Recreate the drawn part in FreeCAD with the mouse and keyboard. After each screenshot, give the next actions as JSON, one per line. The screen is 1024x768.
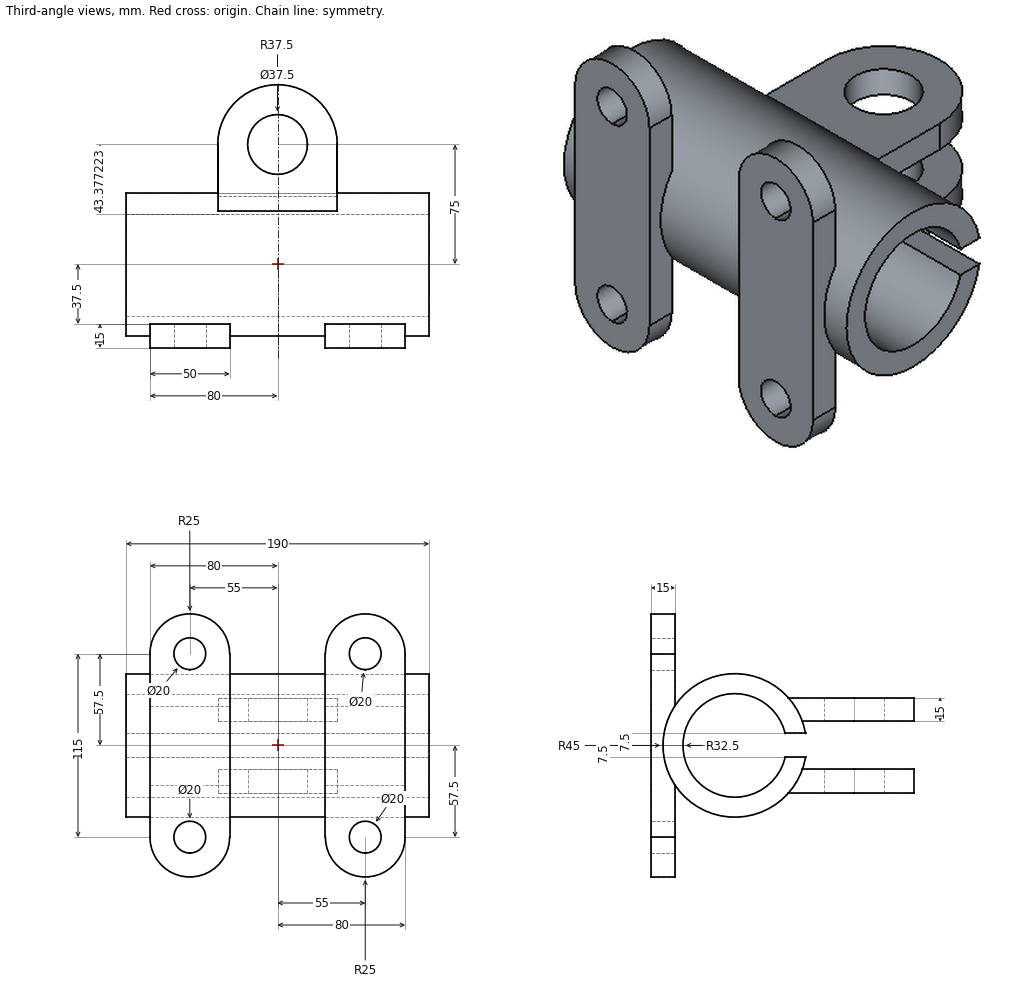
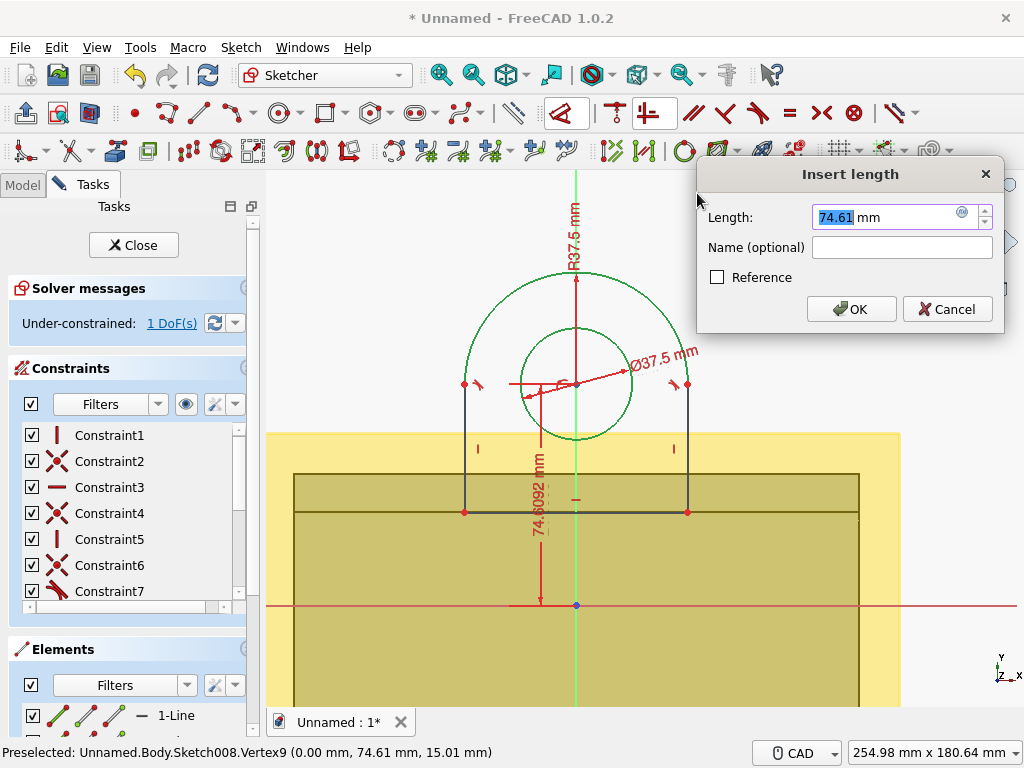
{"action": "type", "text": "75"}
{"action": "key", "text": "Return"}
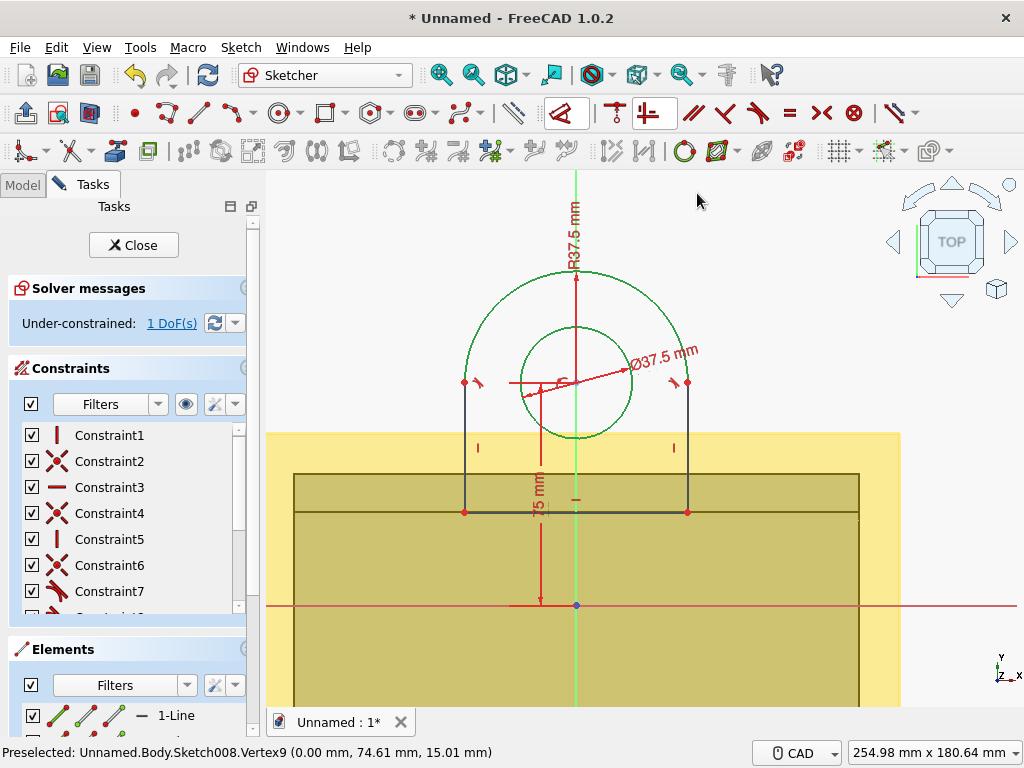
{"action": "left_click", "coordinate": [465, 422]}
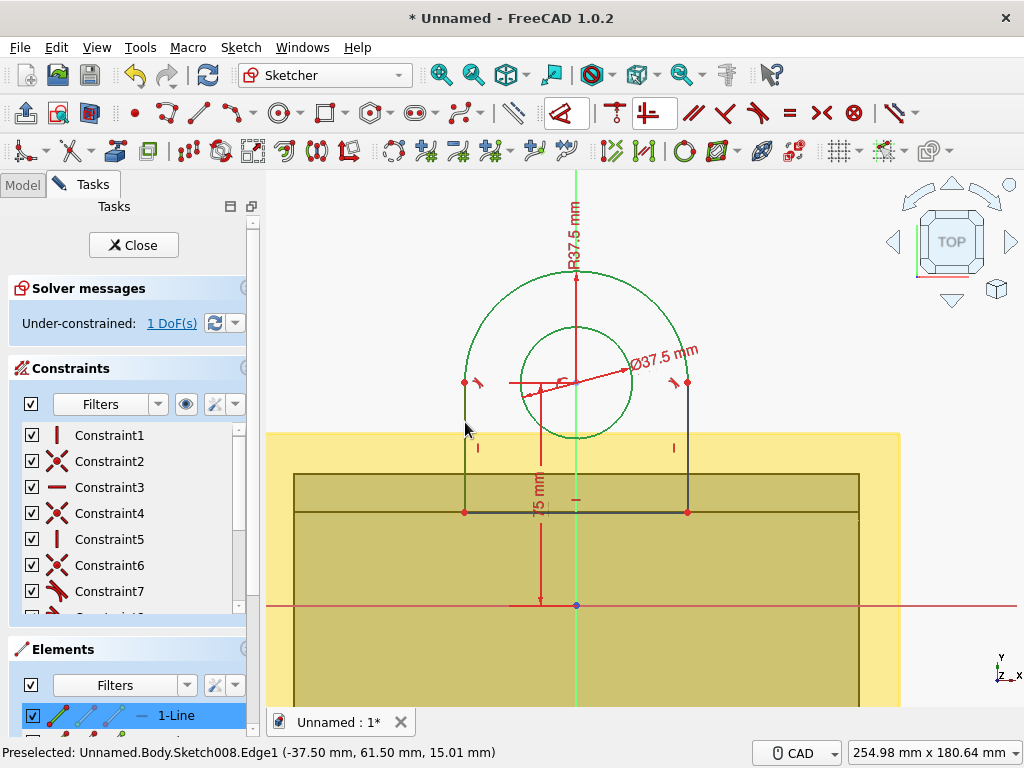
{"action": "left_click", "coordinate": [584, 114]}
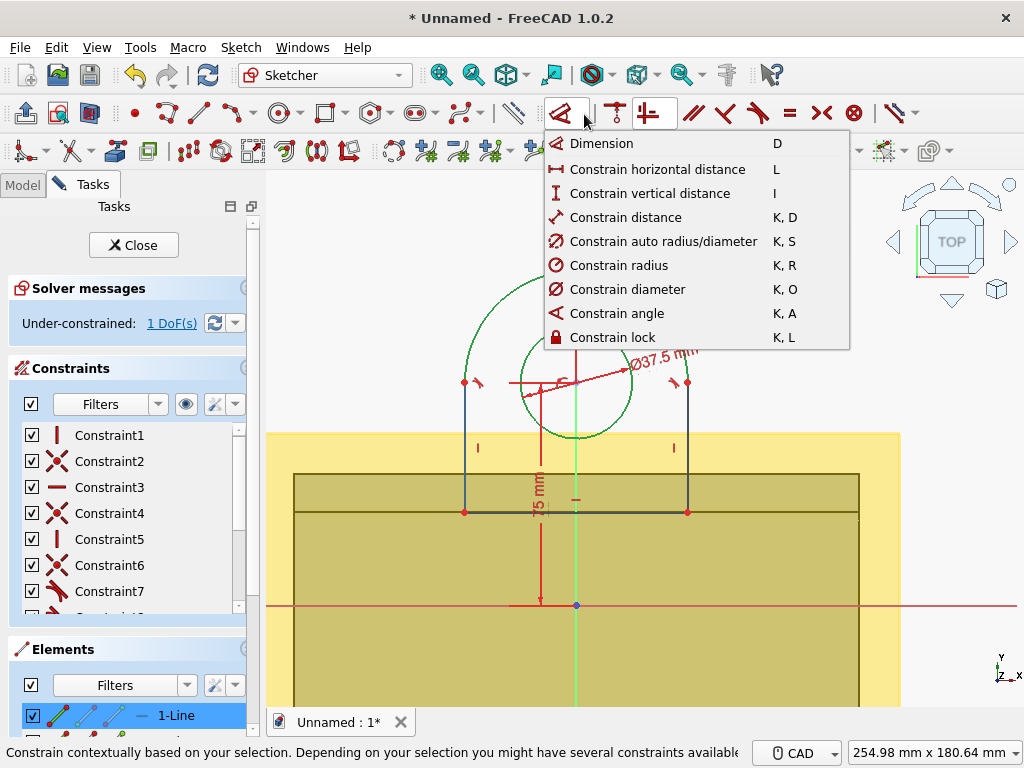
{"action": "left_click", "coordinate": [697, 193]}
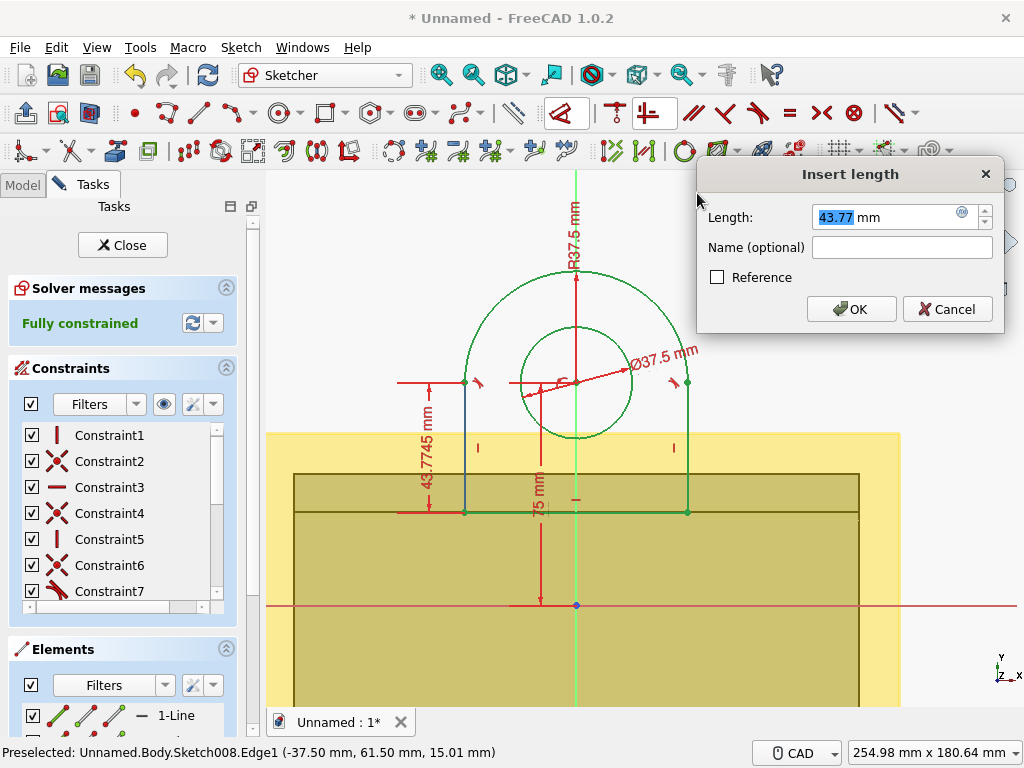
{"action": "type", "text": "43.377223"}
{"action": "key", "text": "Return"}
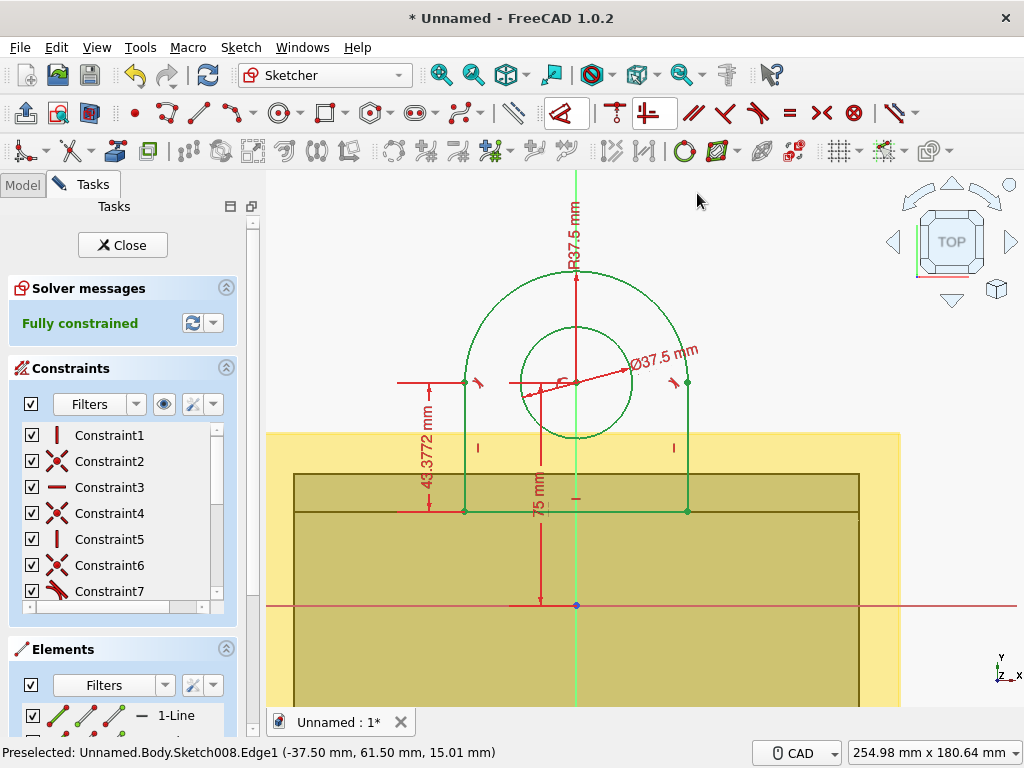
{"action": "left_click", "coordinate": [123, 245]}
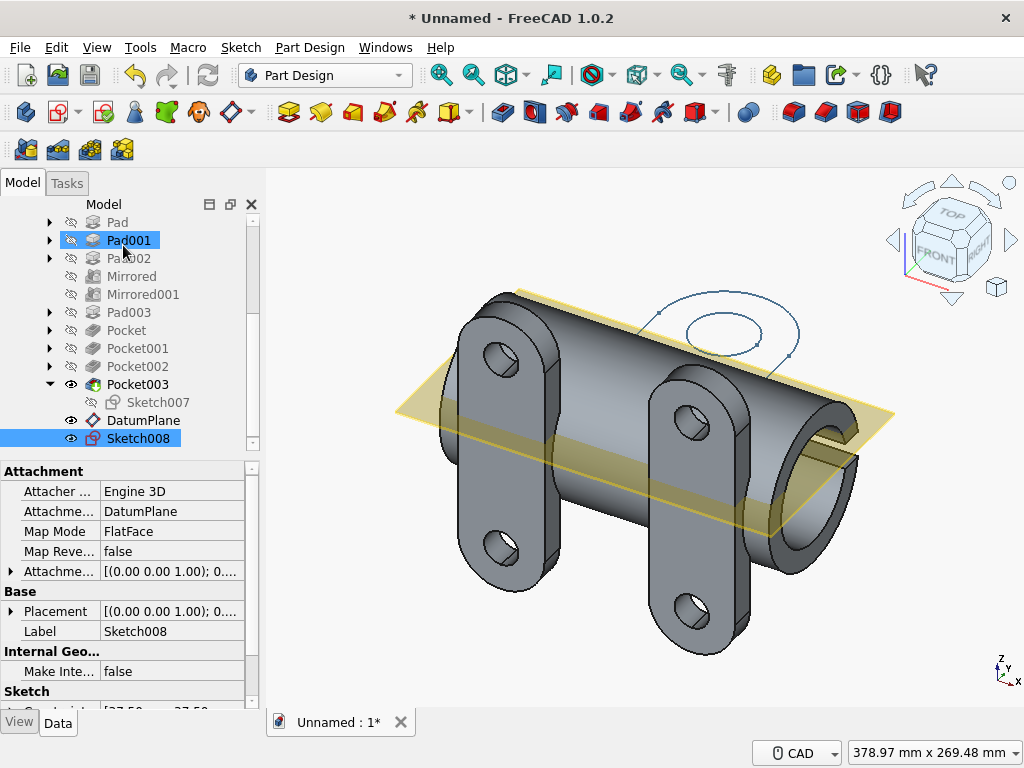
{"action": "left_click", "coordinate": [290, 112]}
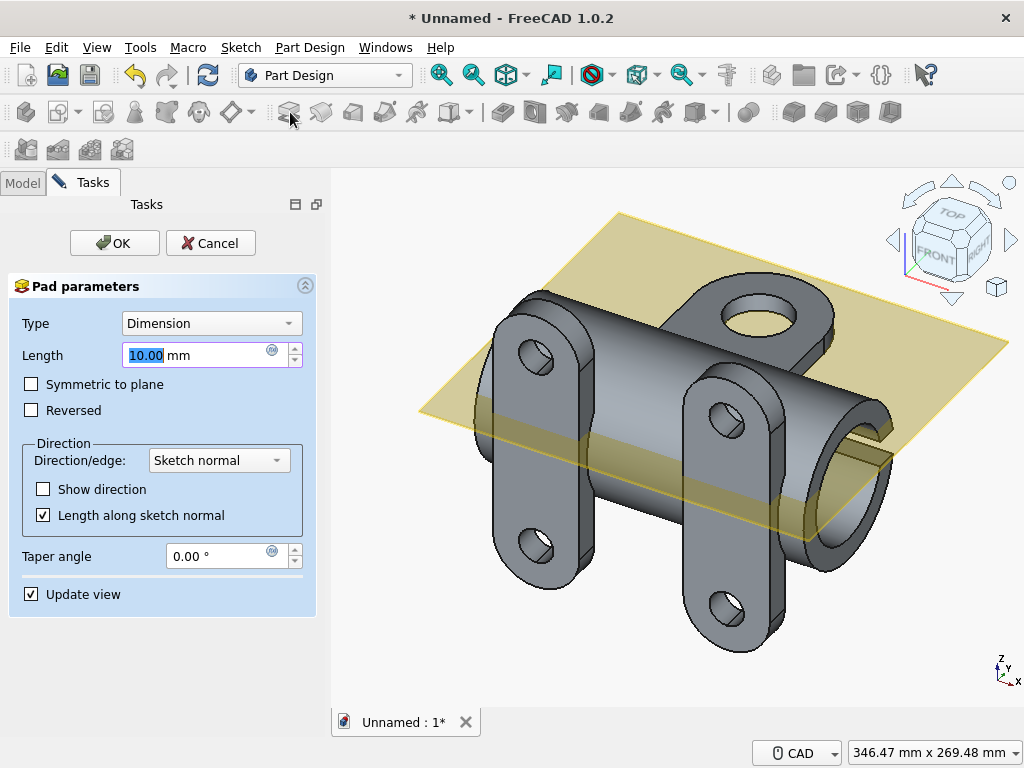
{"action": "type", "text": "15"}
{"action": "key", "text": "Tab"}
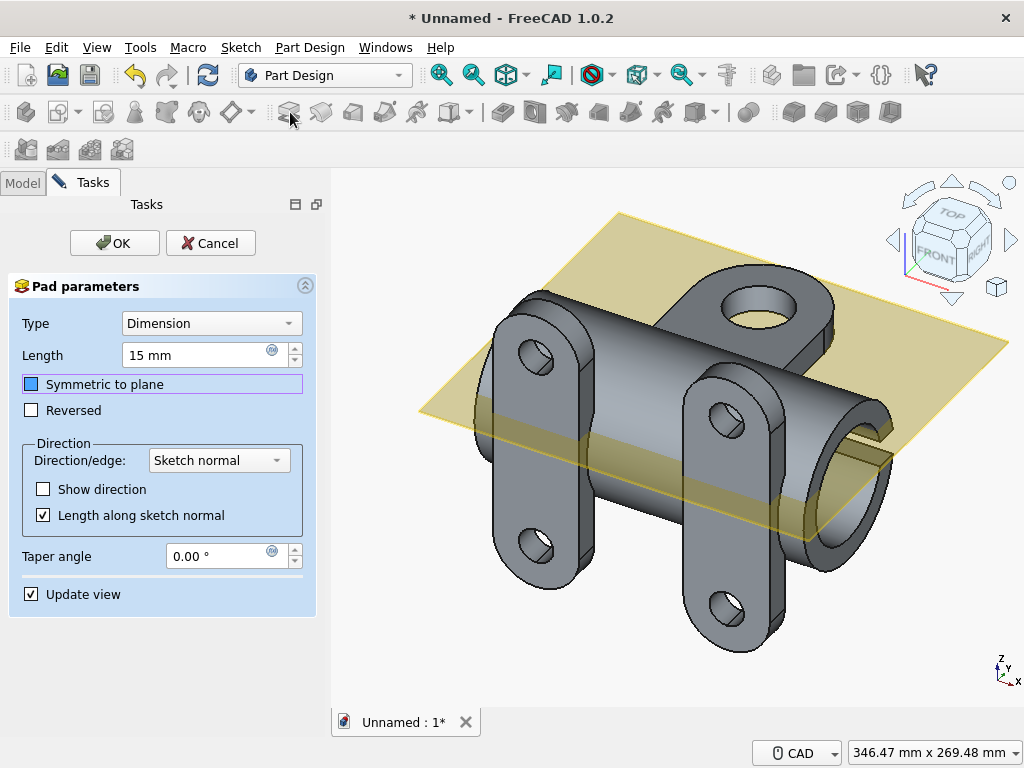
{"action": "left_click", "coordinate": [115, 243]}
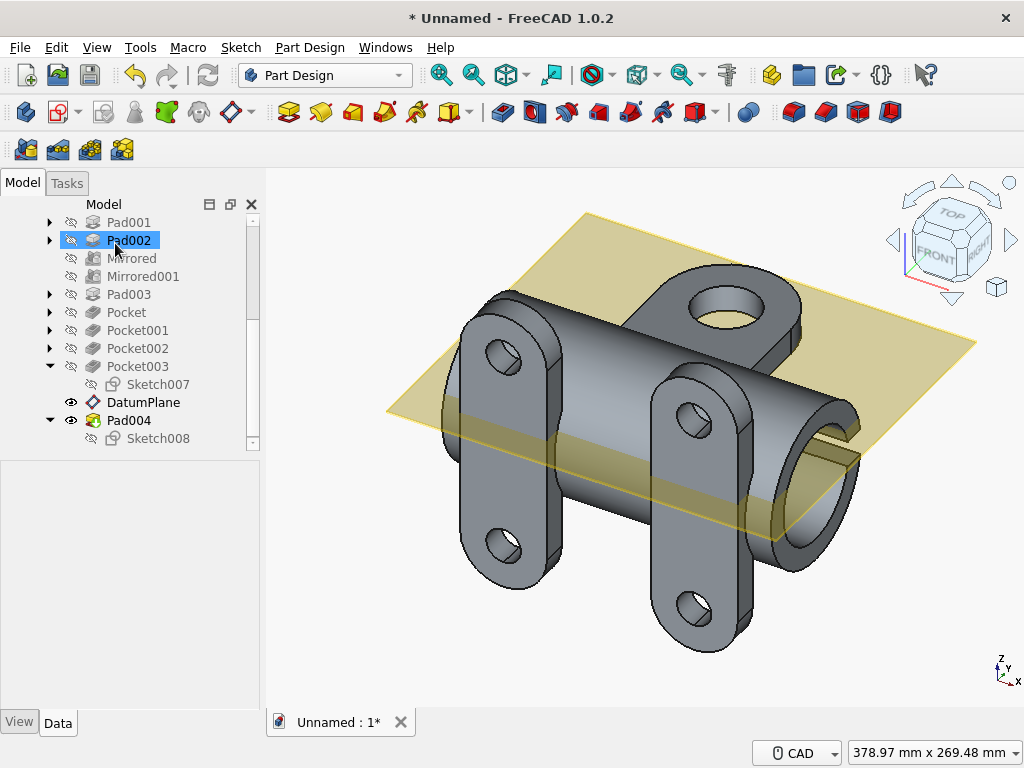
{"action": "left_click", "coordinate": [116, 402]}
{"action": "key", "text": "space"}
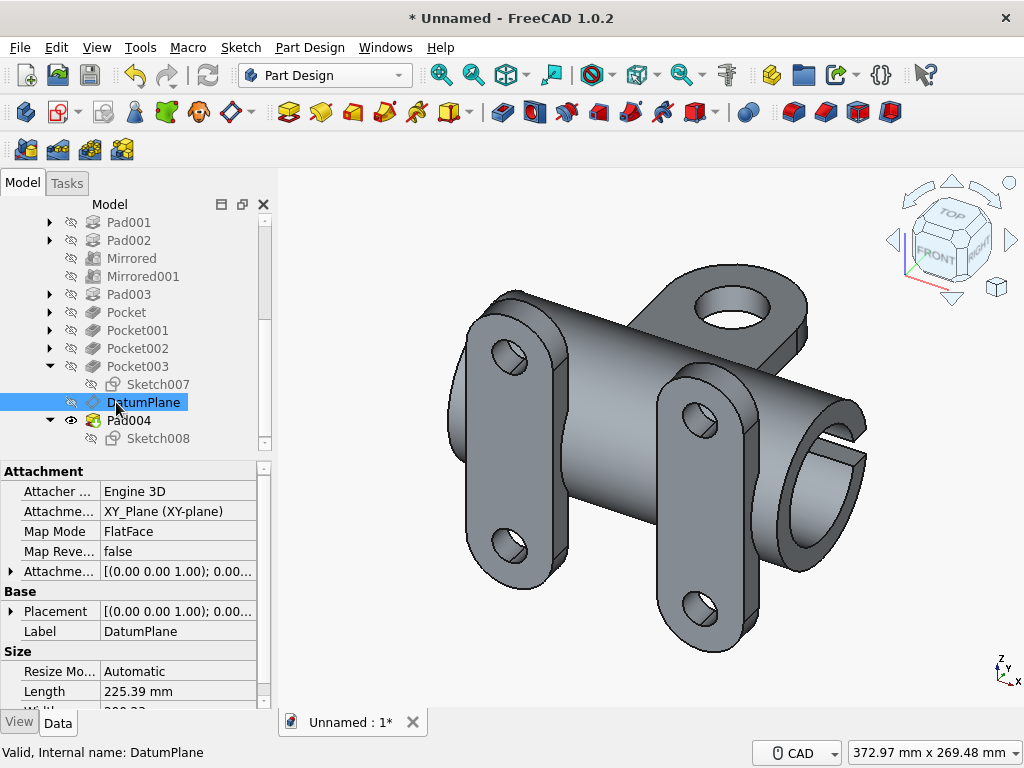
{"action": "left_click", "coordinate": [442, 76]}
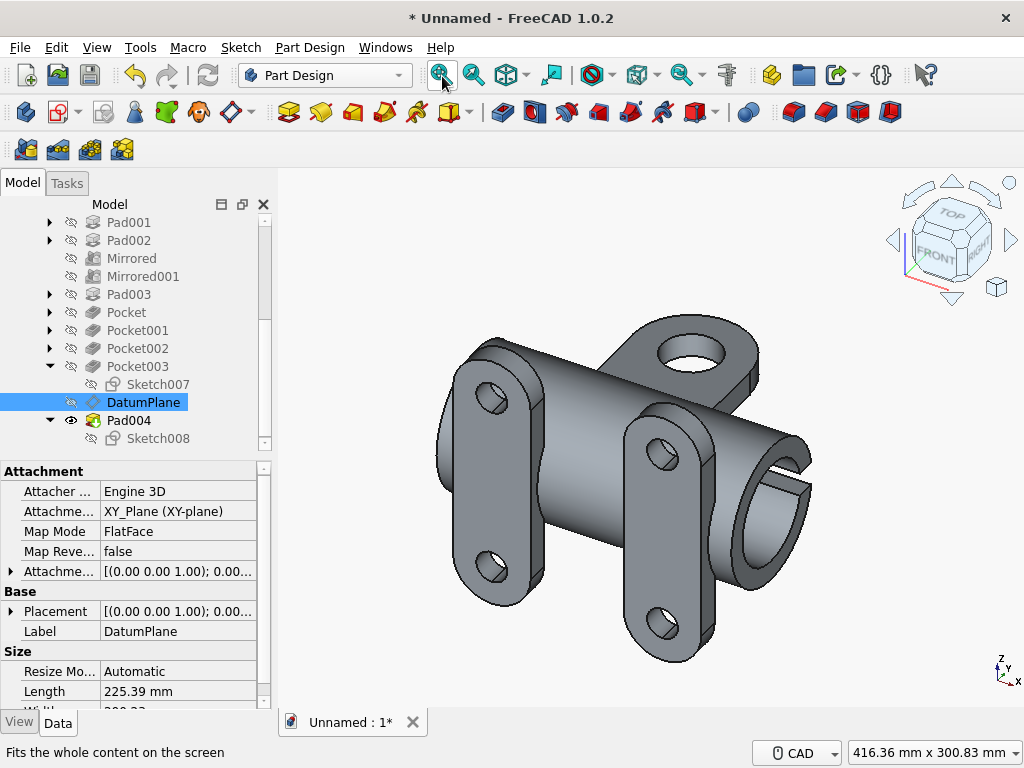
{"action": "left_click", "coordinate": [116, 420]}